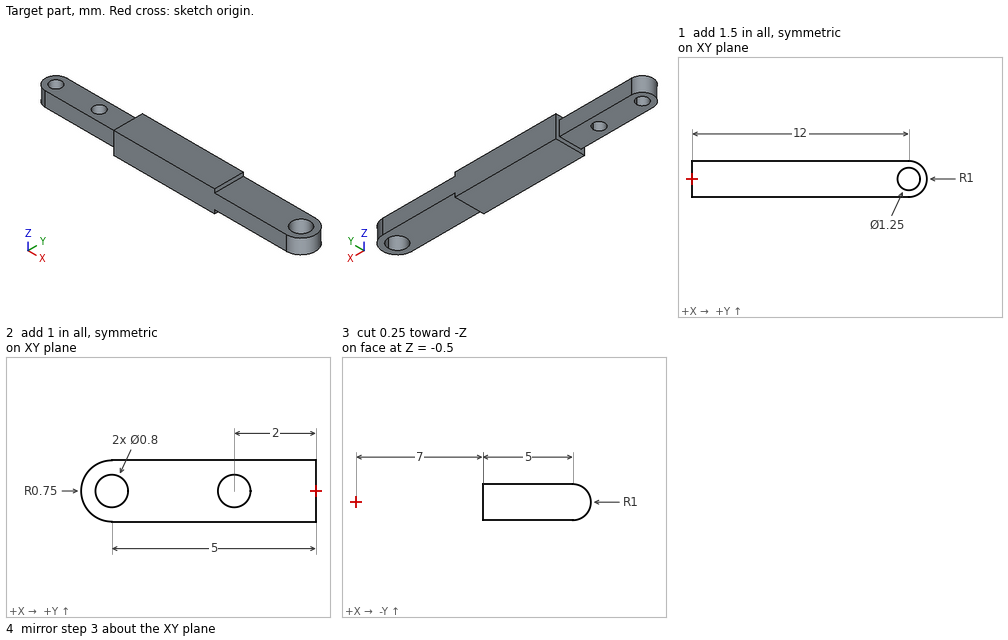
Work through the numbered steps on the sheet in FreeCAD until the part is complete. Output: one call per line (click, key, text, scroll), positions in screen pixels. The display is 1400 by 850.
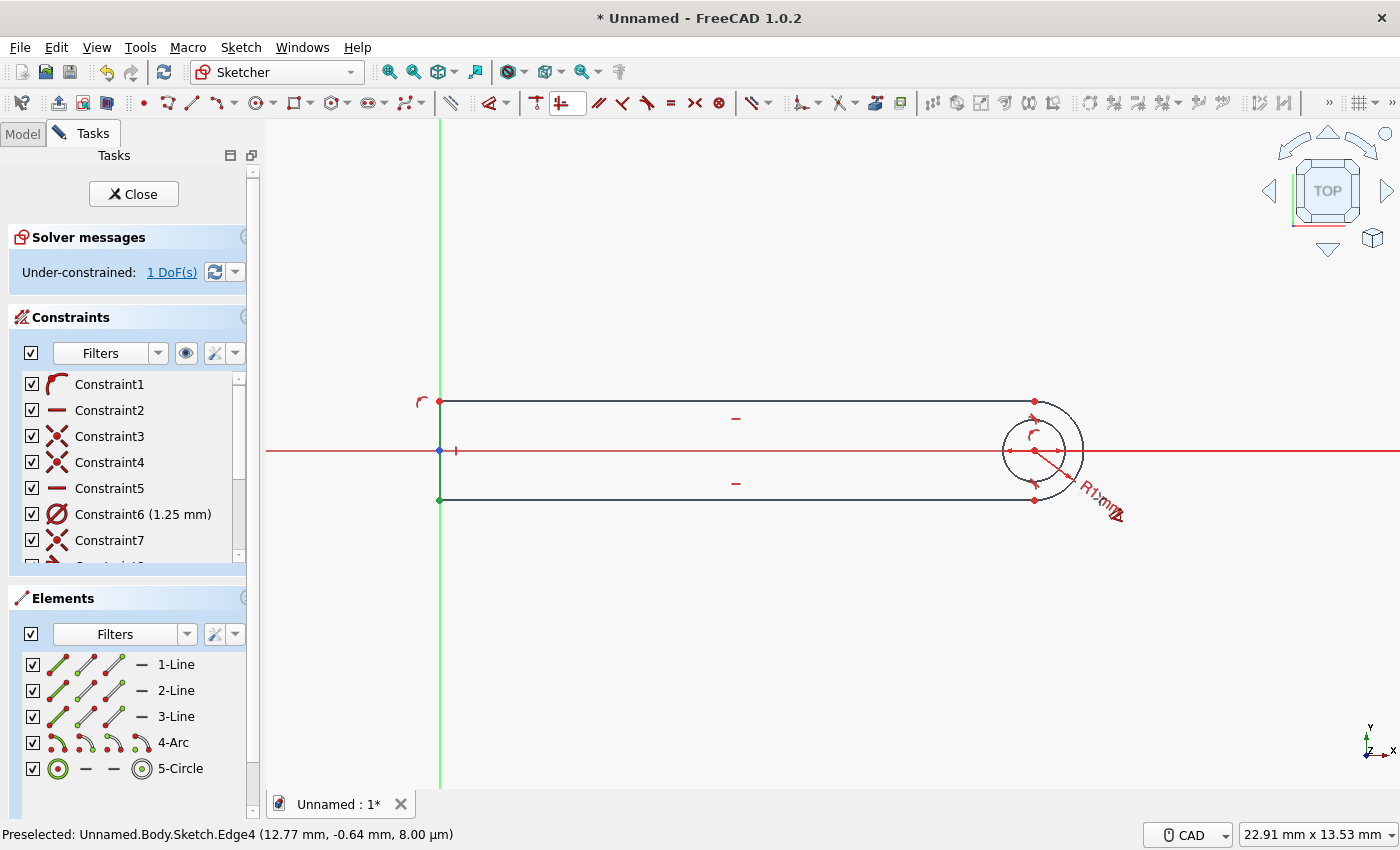
click(856, 401)
click(737, 367)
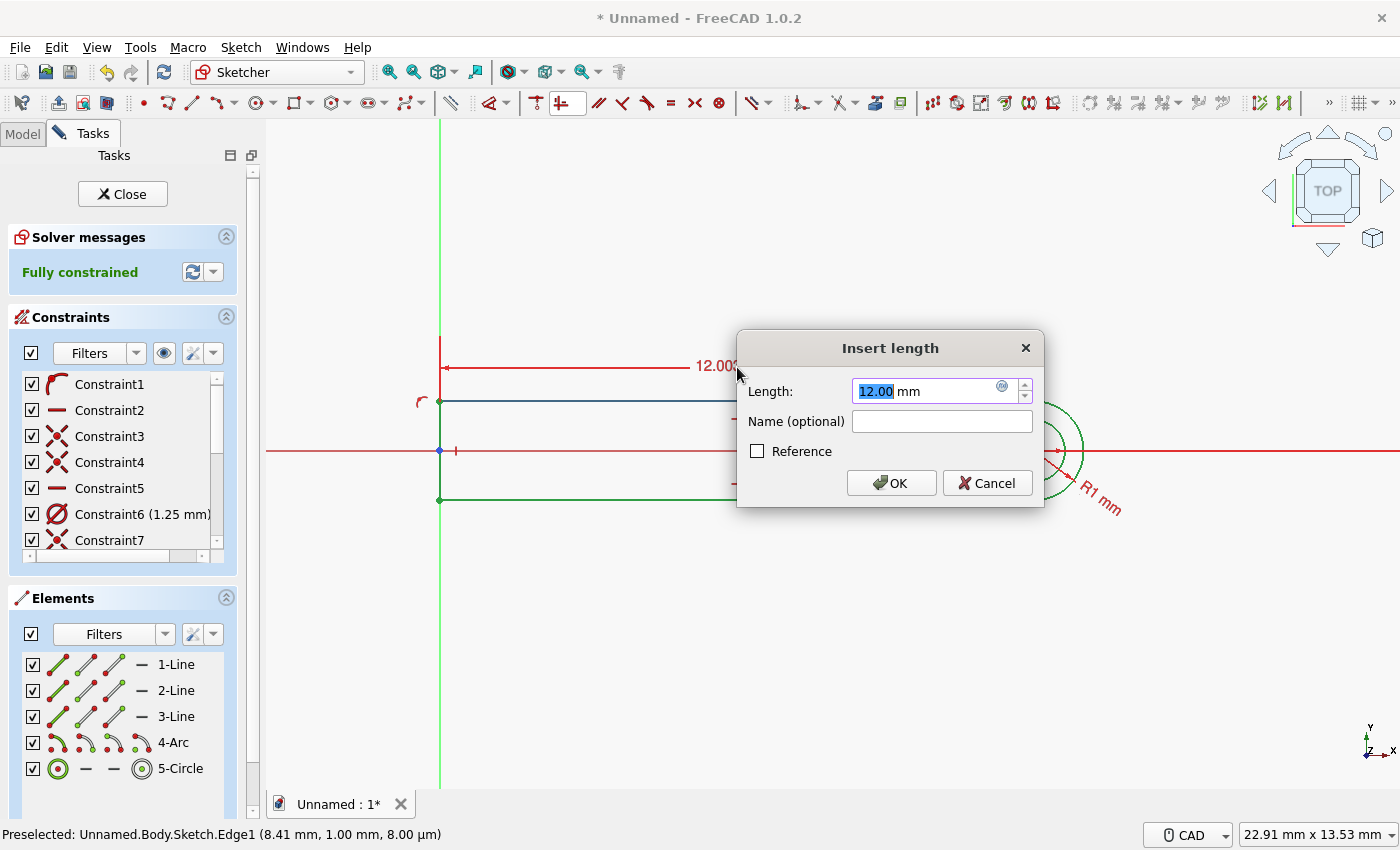
text(12)
key(Return)
key(Escape)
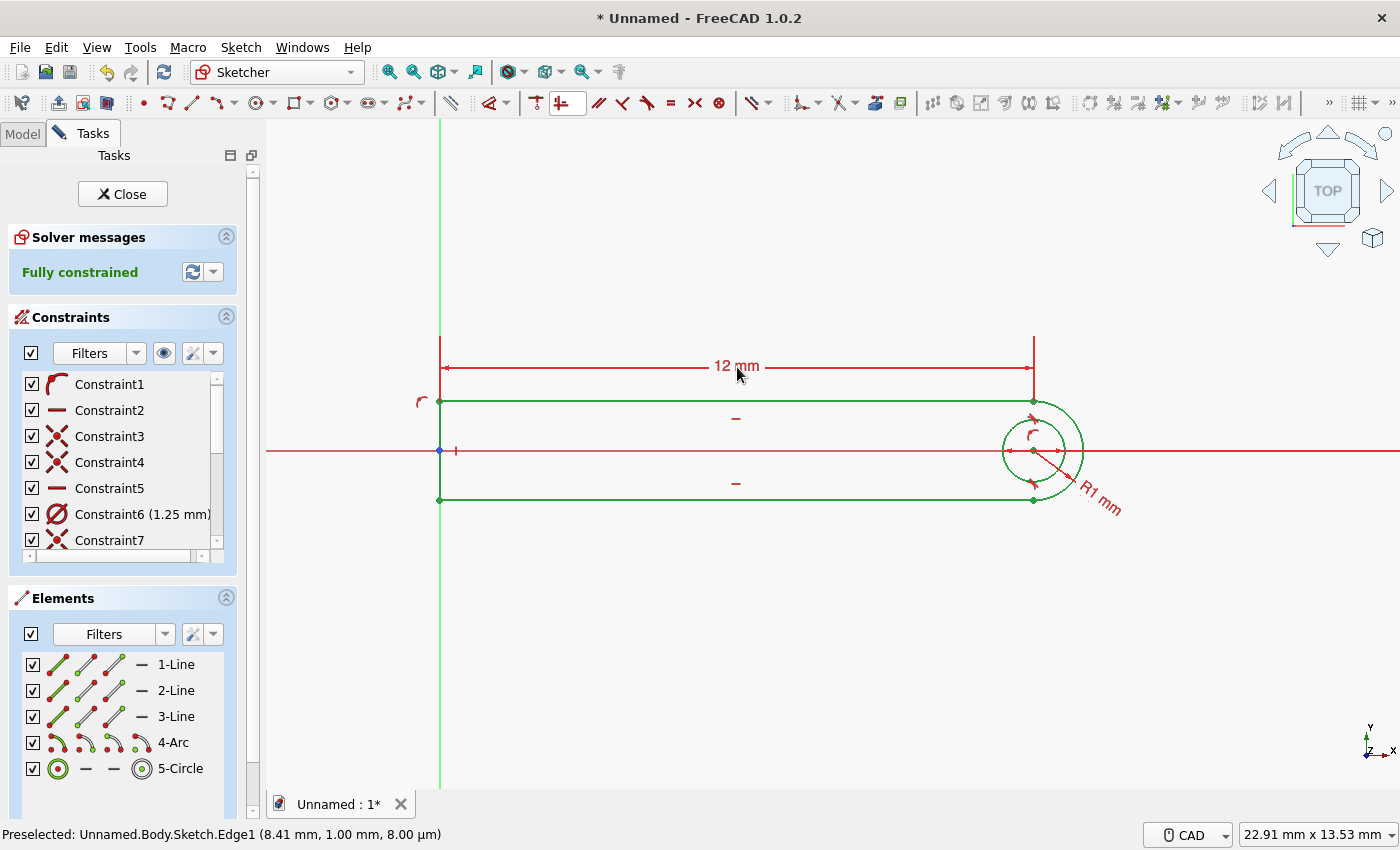
click(123, 194)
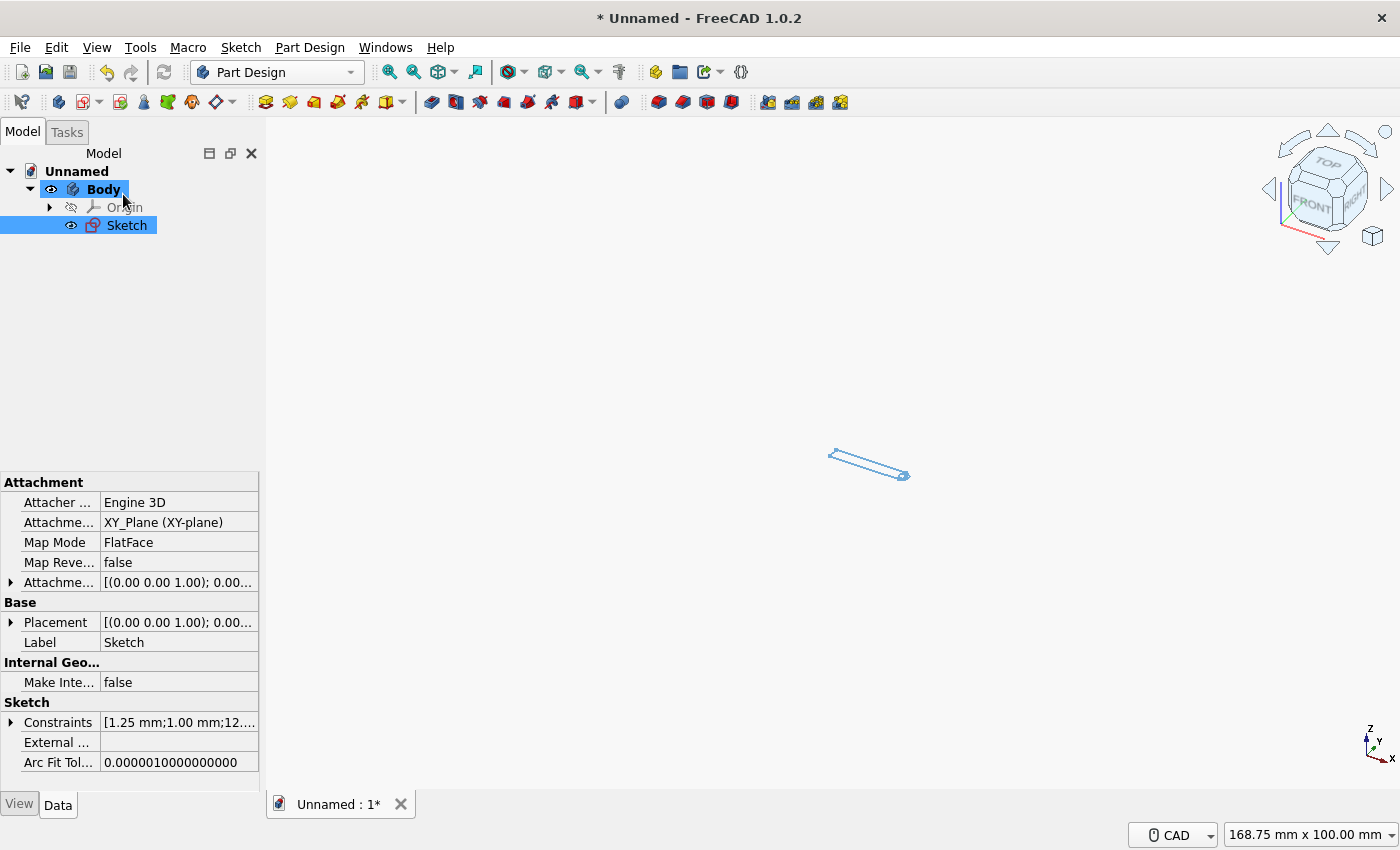
click(266, 102)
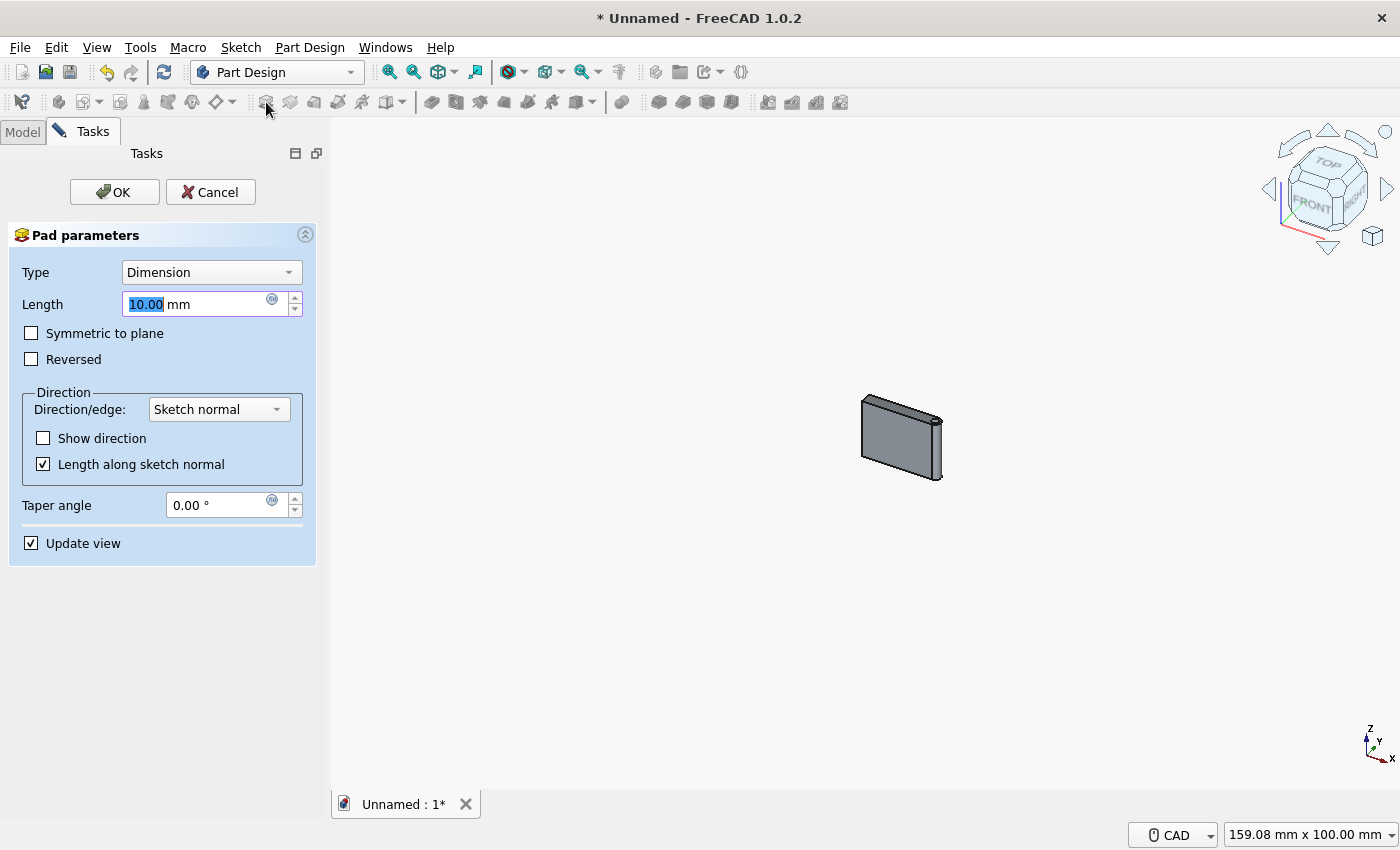
text(1.5)
key(Tab)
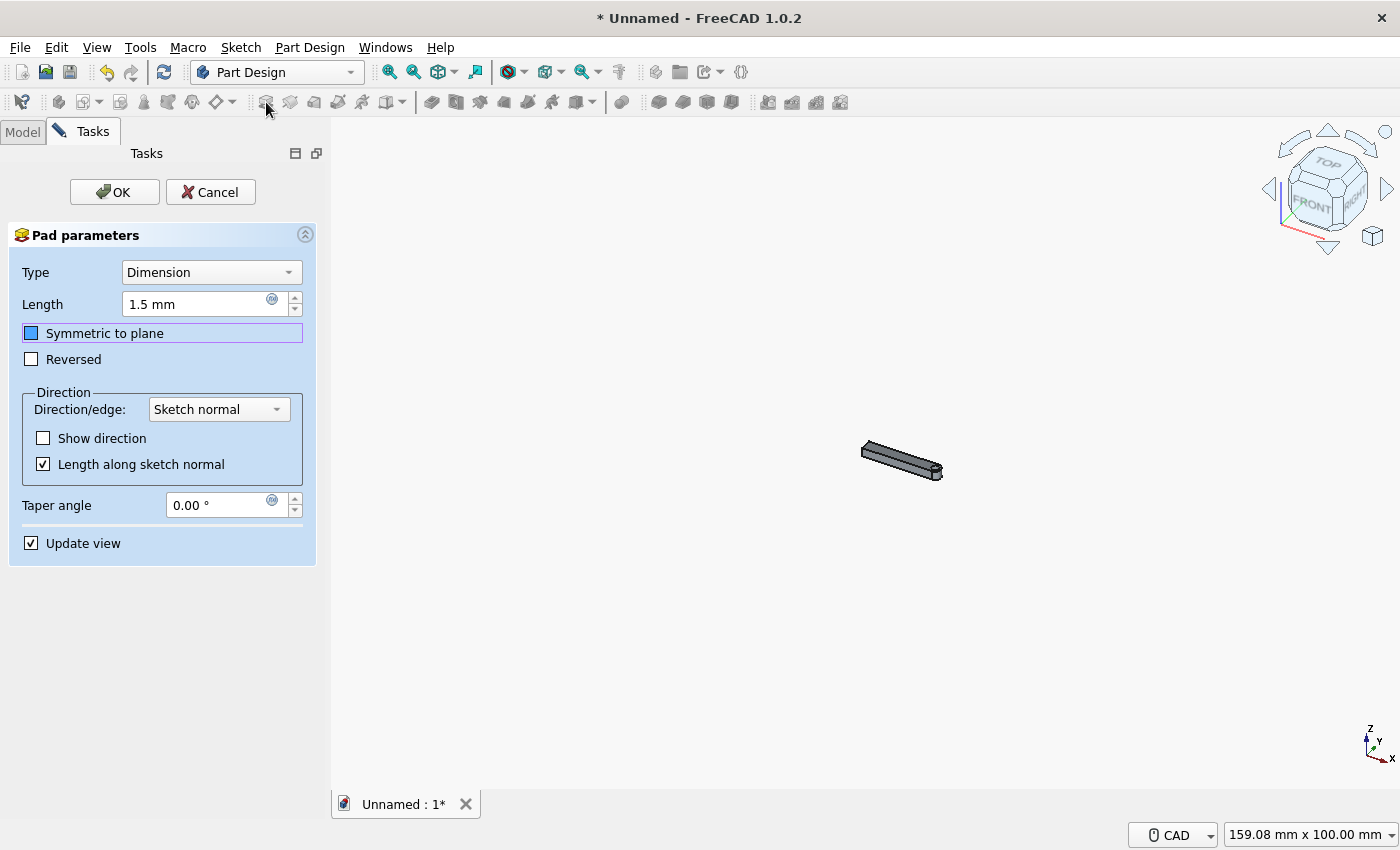
click(30, 333)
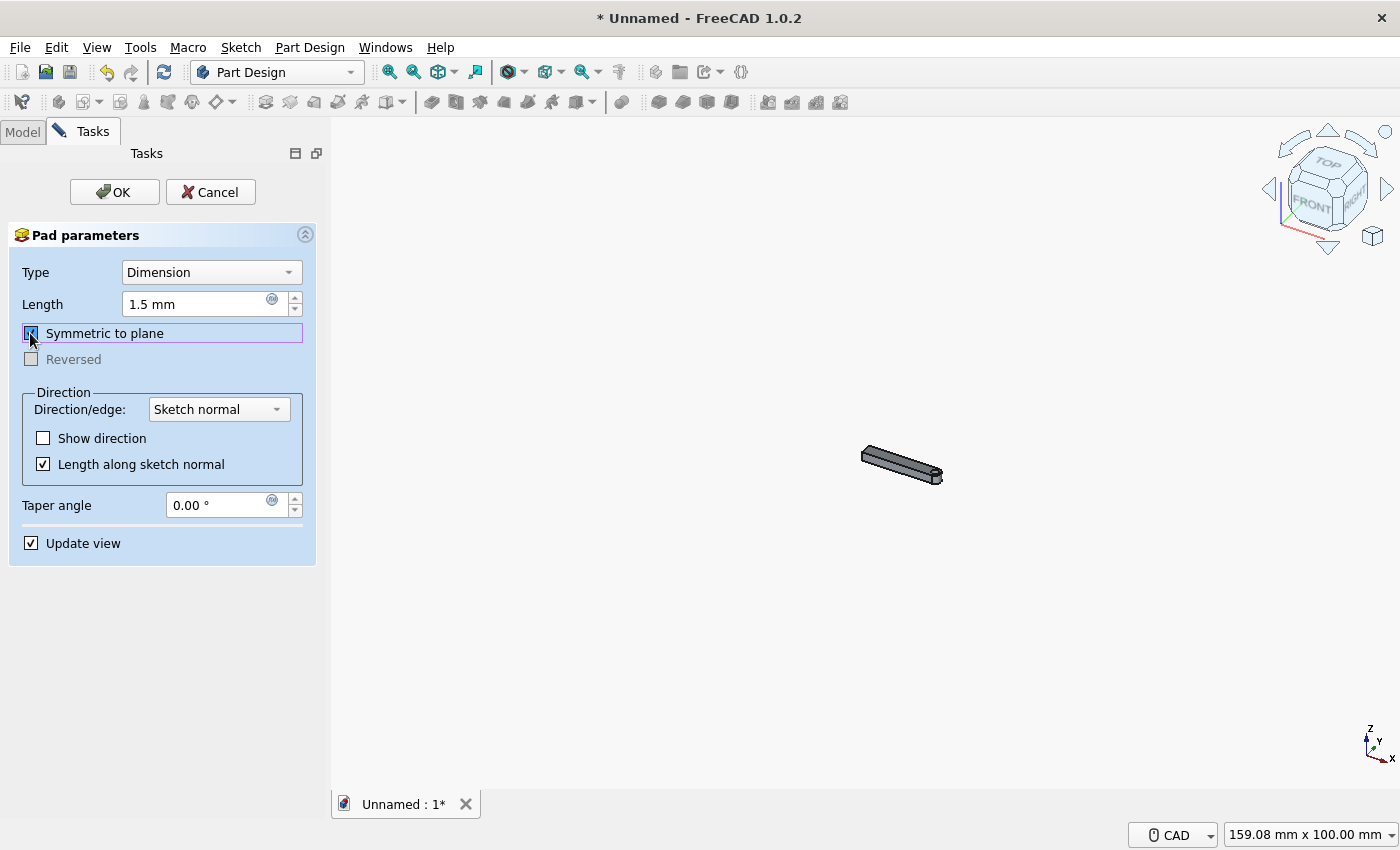
click(115, 192)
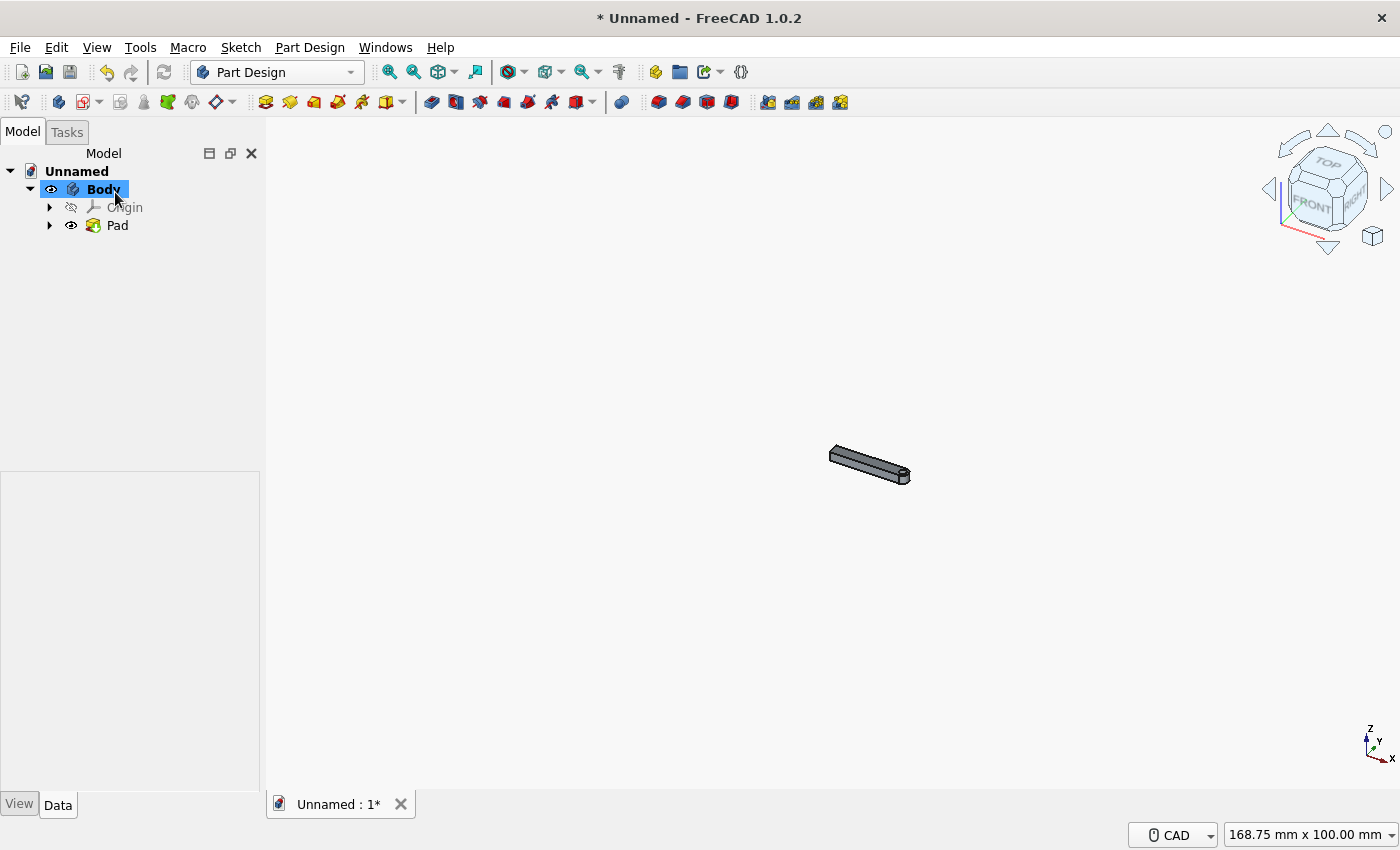
key(v)
key(f)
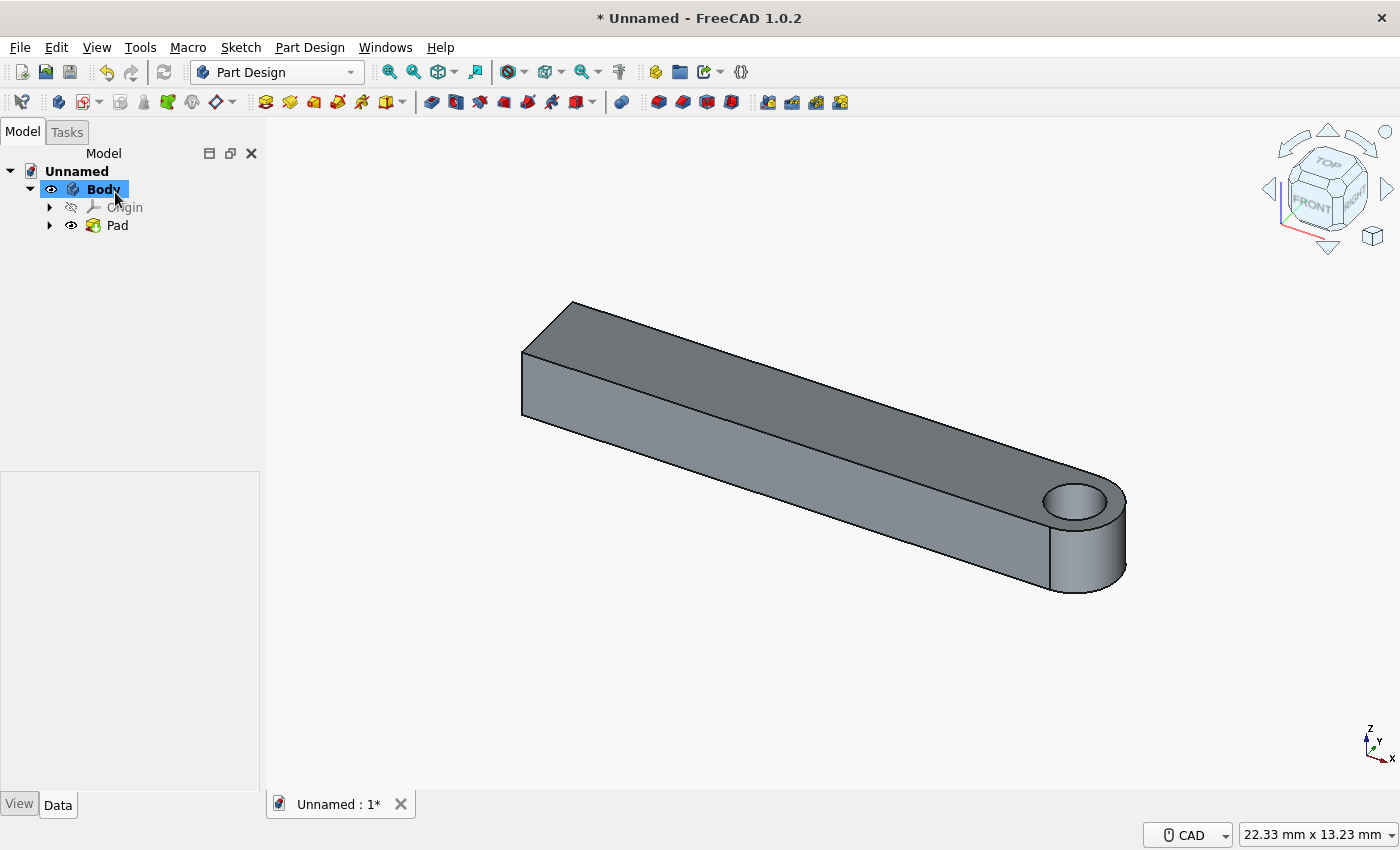
click(84, 102)